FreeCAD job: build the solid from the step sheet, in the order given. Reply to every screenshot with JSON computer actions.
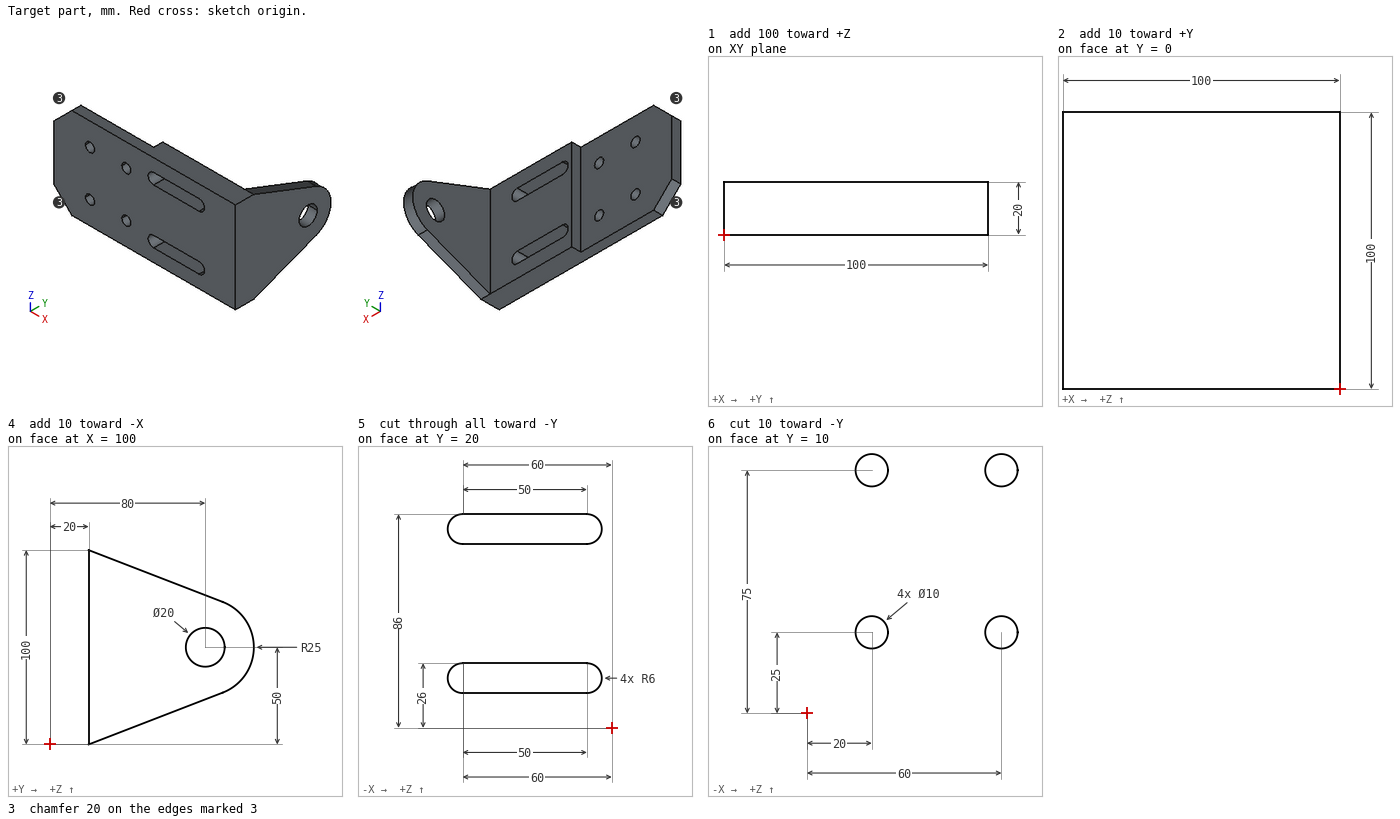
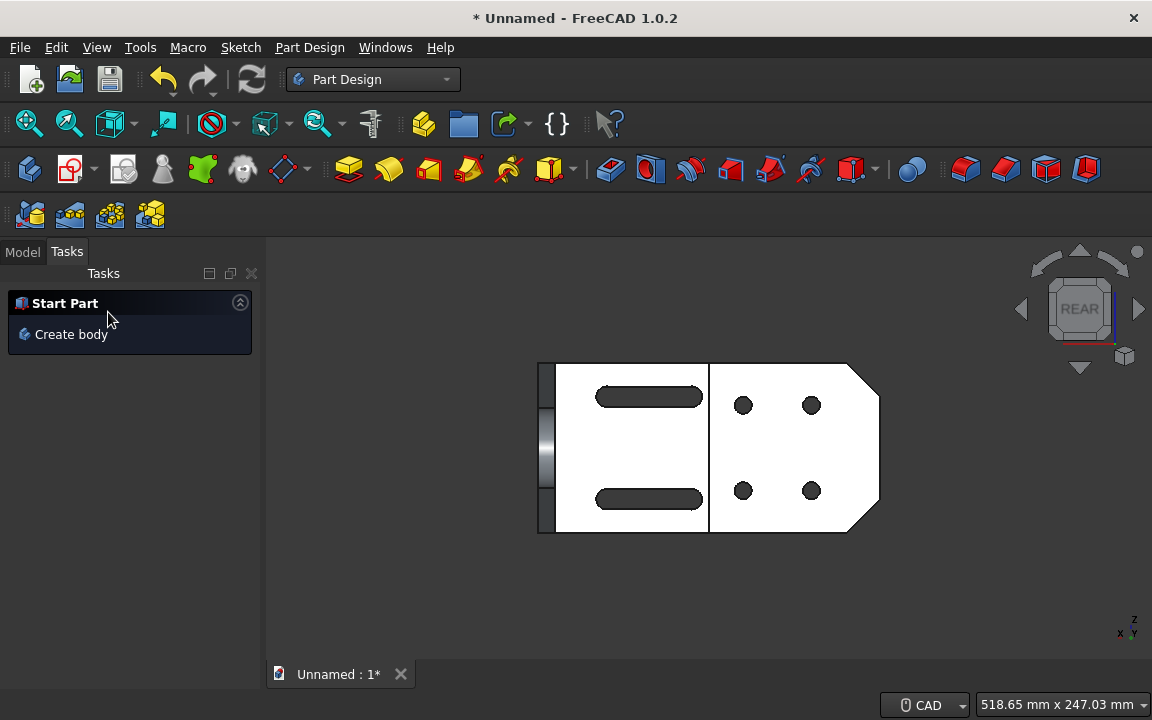
{"action": "key", "text": "0"}